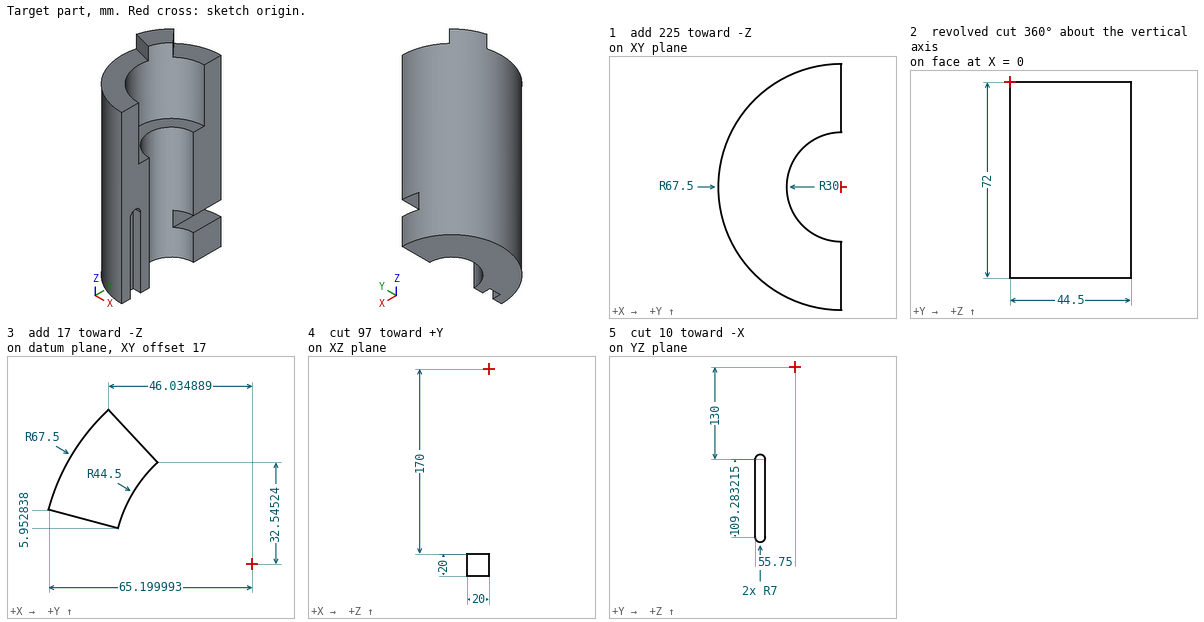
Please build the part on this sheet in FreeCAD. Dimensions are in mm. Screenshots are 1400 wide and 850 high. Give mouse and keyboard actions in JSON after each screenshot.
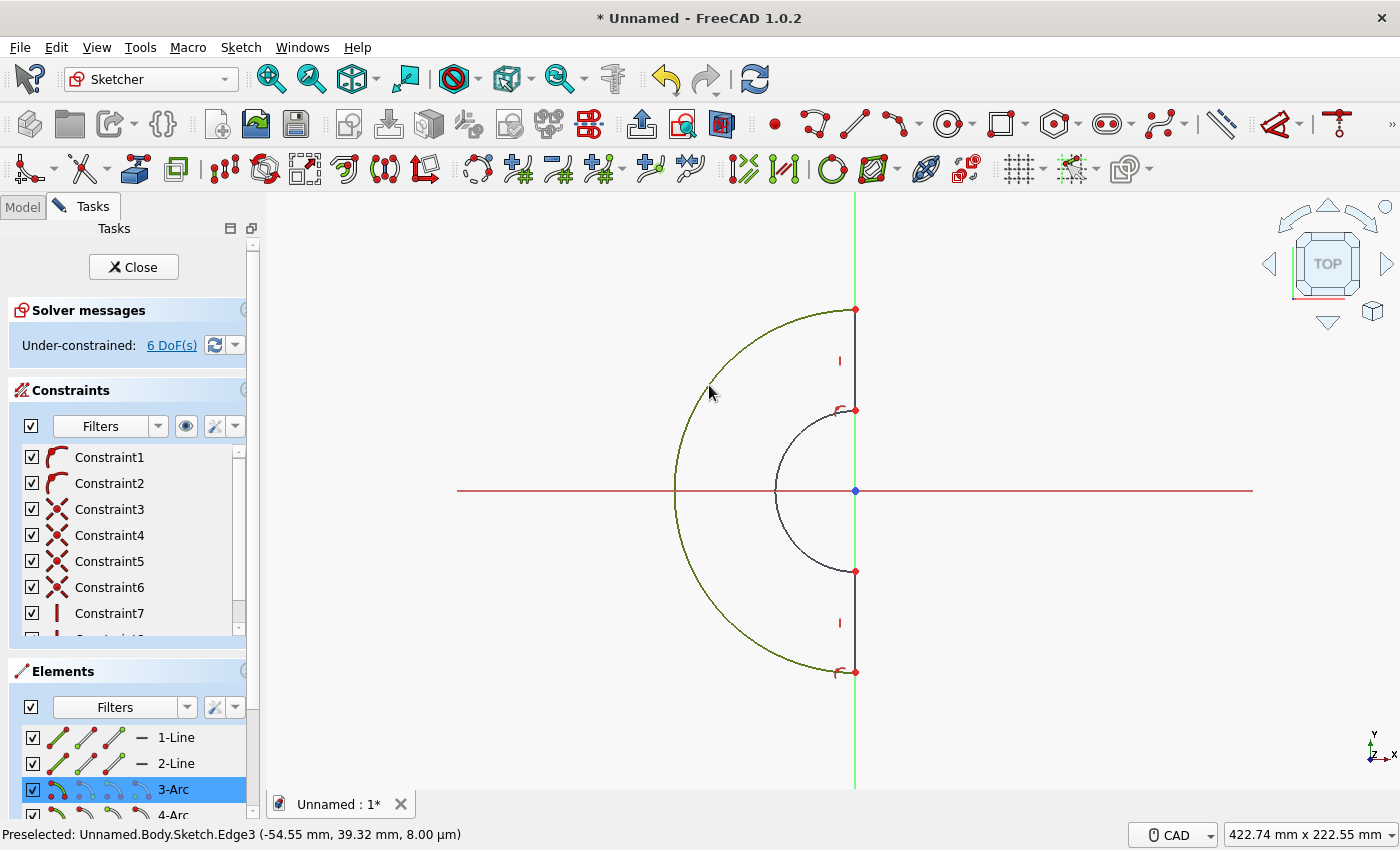
{"action": "left_click", "coordinate": [791, 444]}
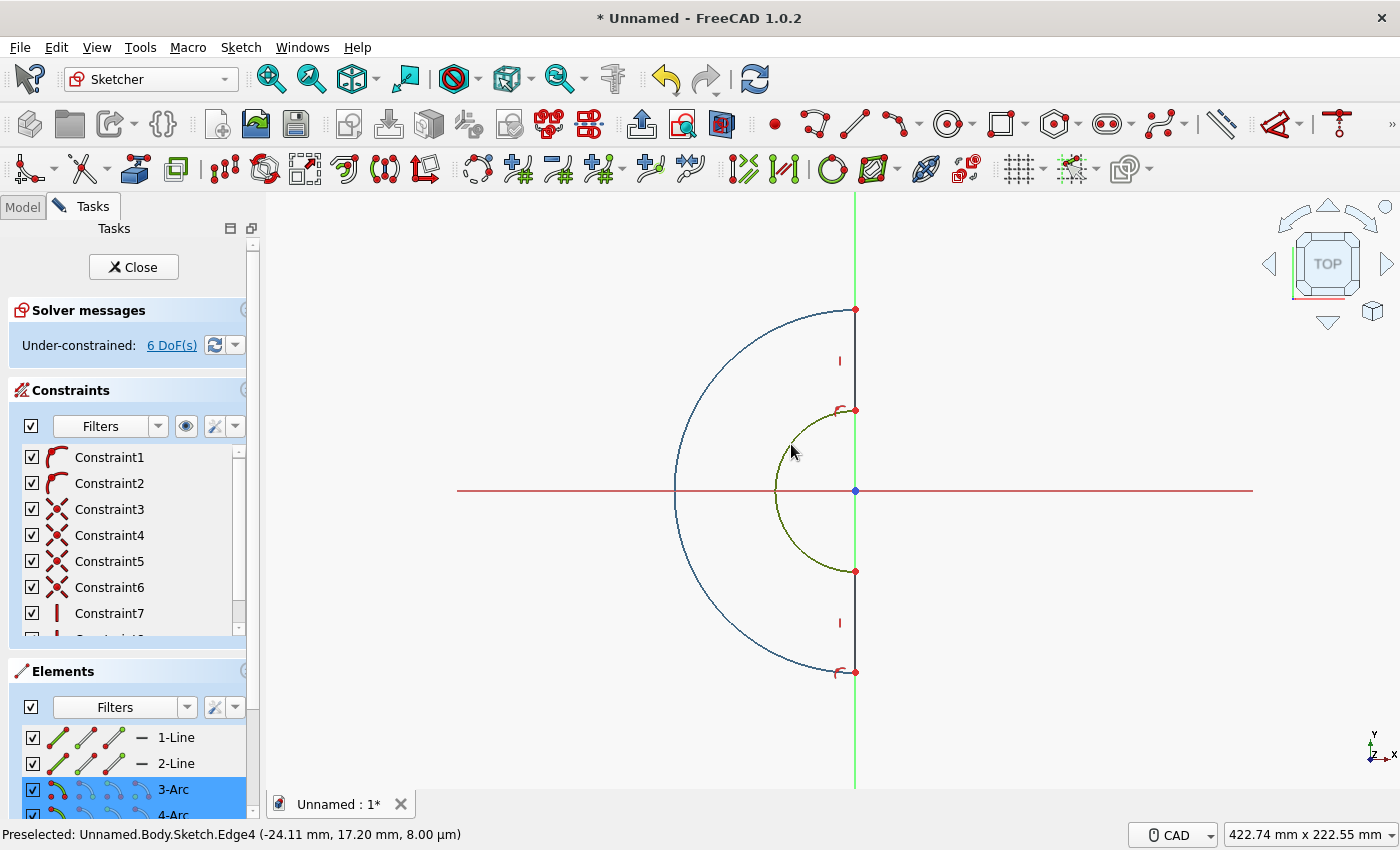
{"action": "left_click", "coordinate": [1338, 124]}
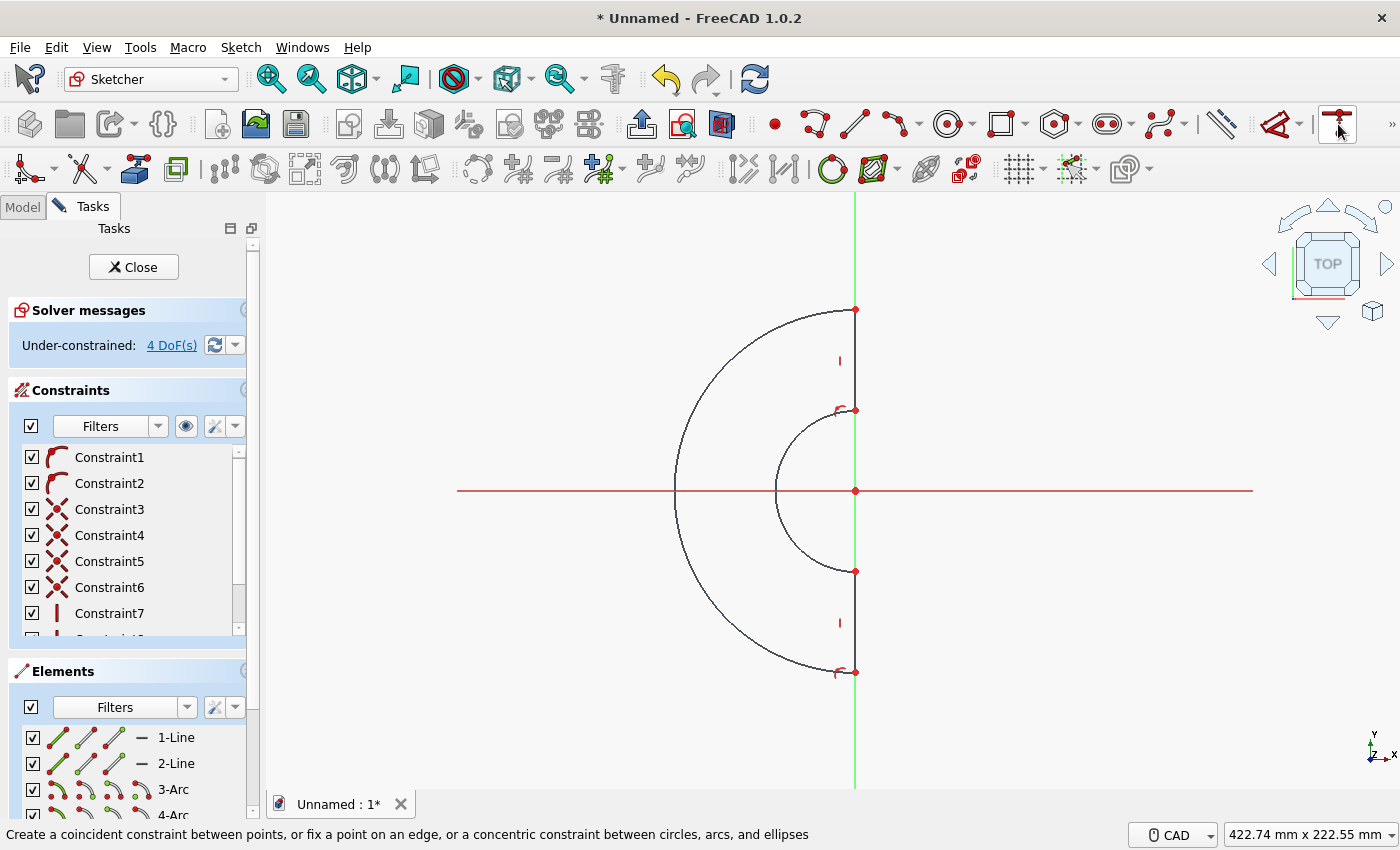
{"action": "left_click_drag", "start_coordinate": [845, 480], "coordinate": [866, 502]}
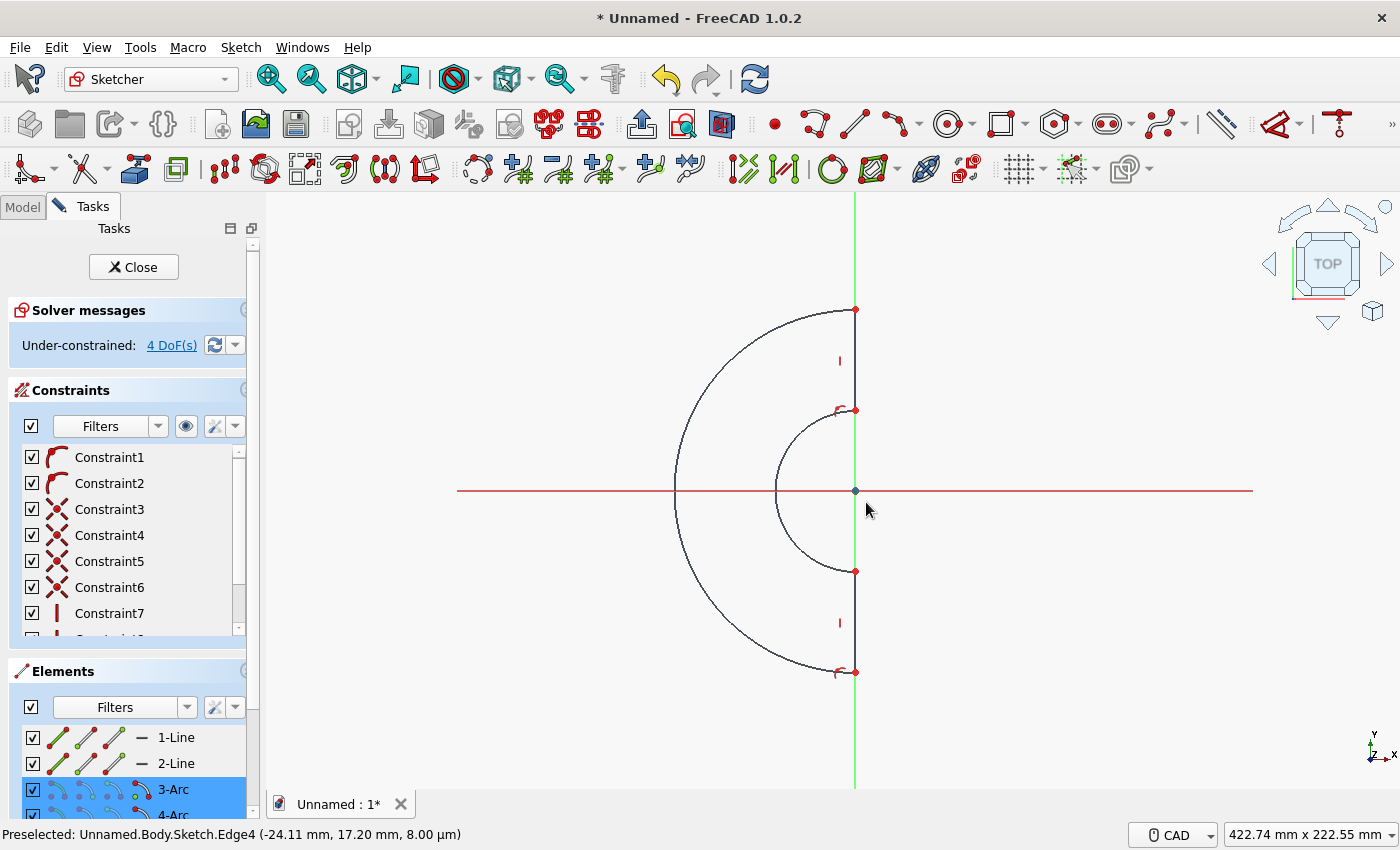
{"action": "left_click", "coordinate": [1338, 124]}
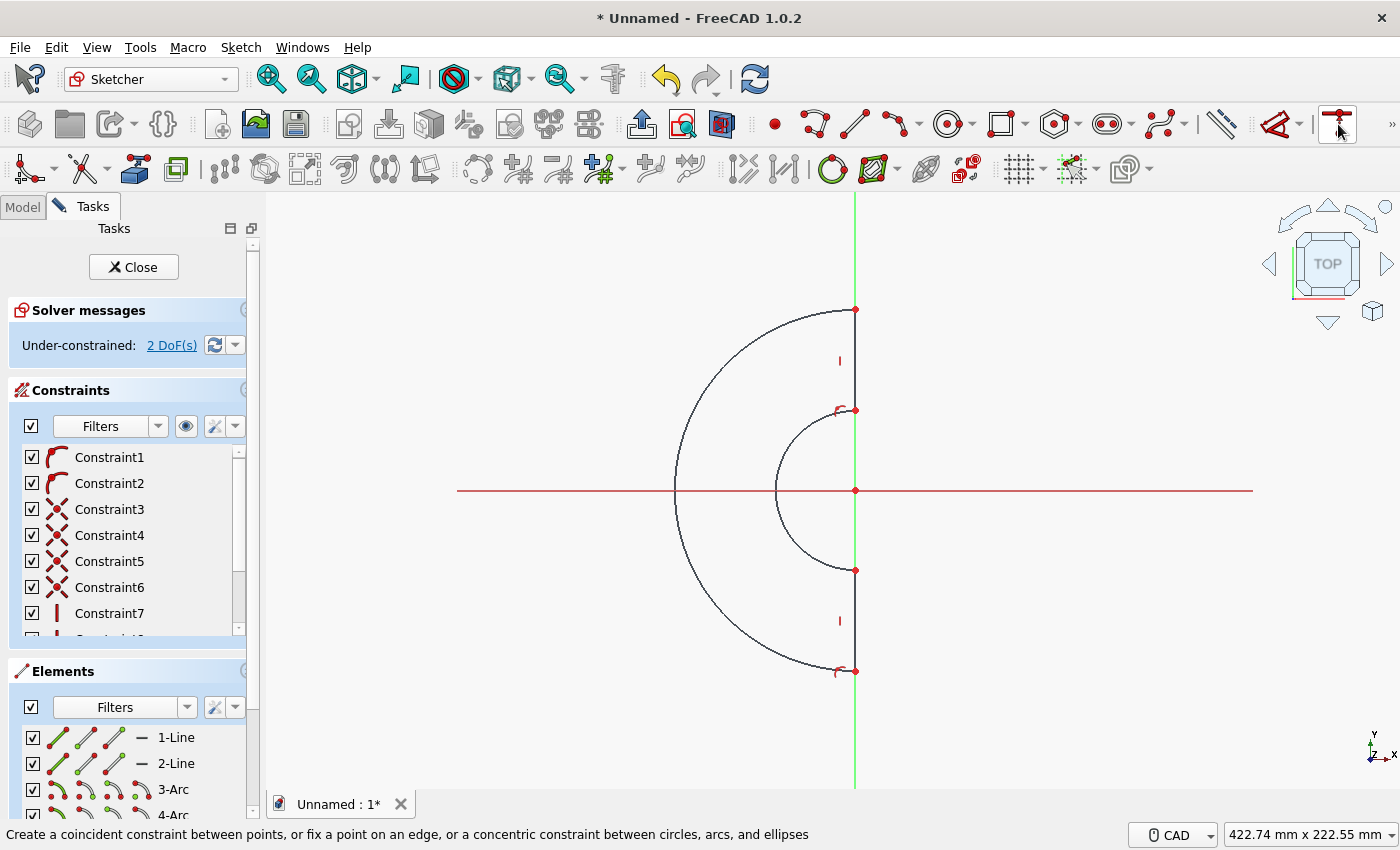
{"action": "left_click", "coordinate": [709, 384]}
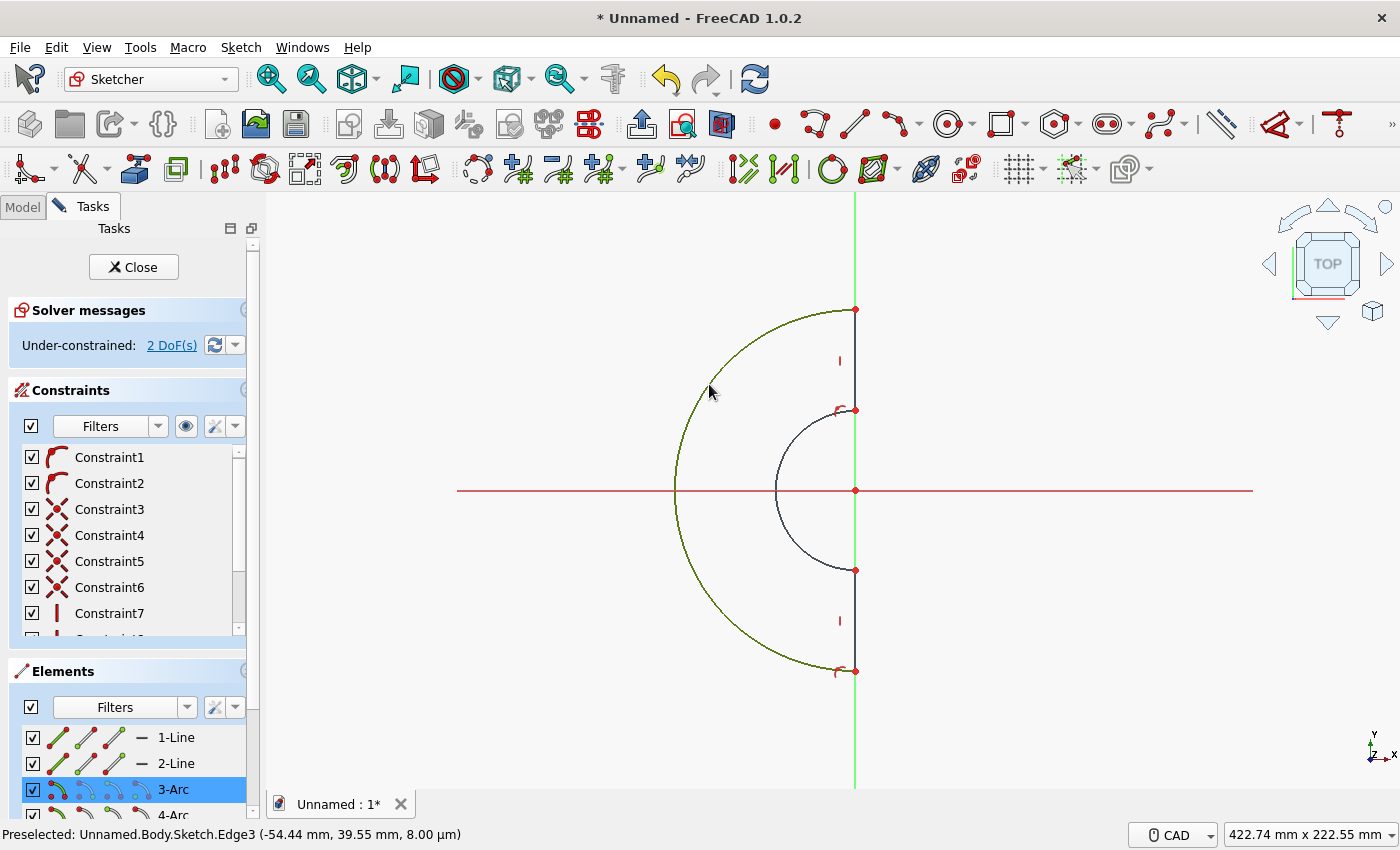
{"action": "key", "text": "k r"}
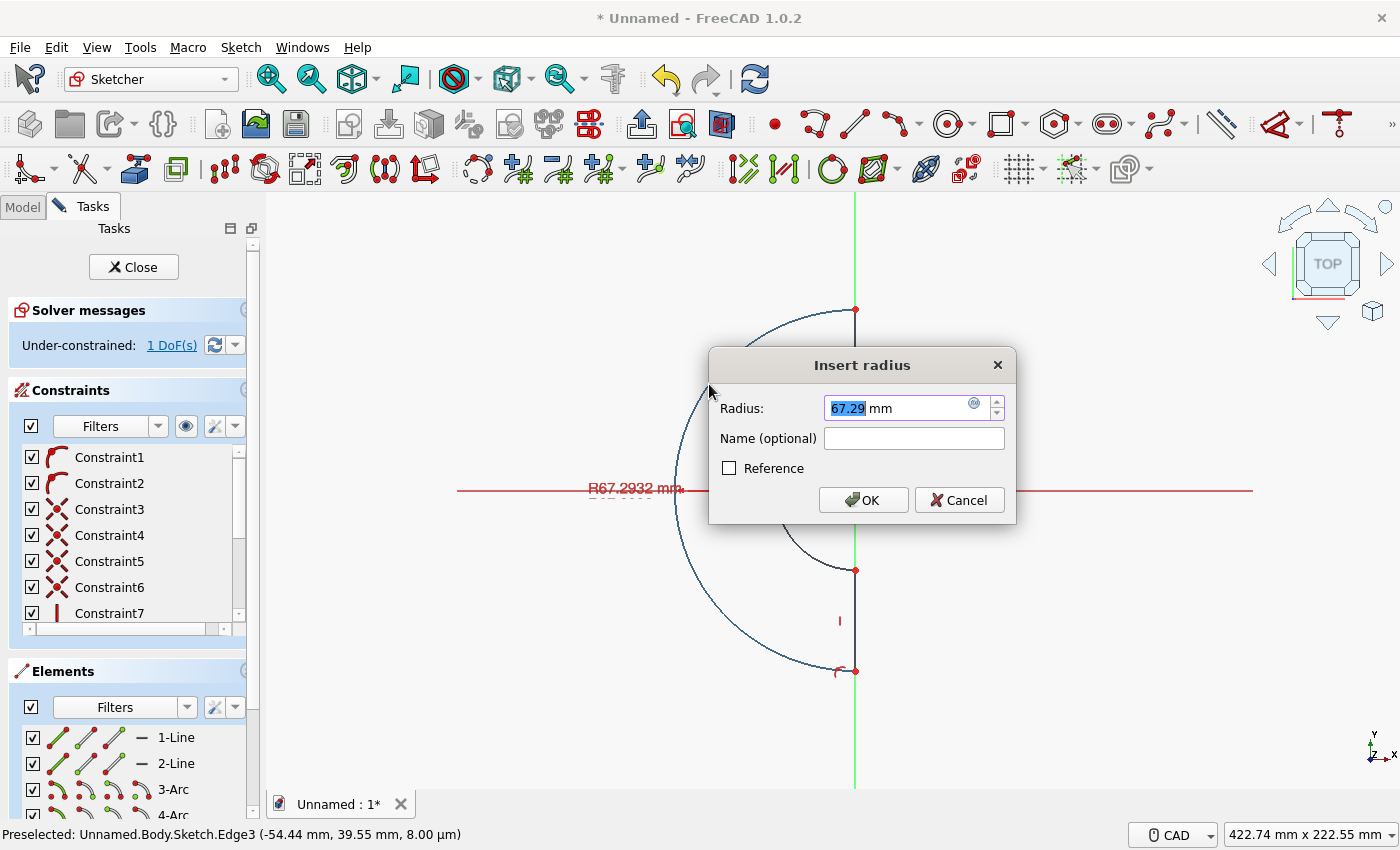
{"action": "type", "text": "67.5"}
{"action": "key", "text": "Return"}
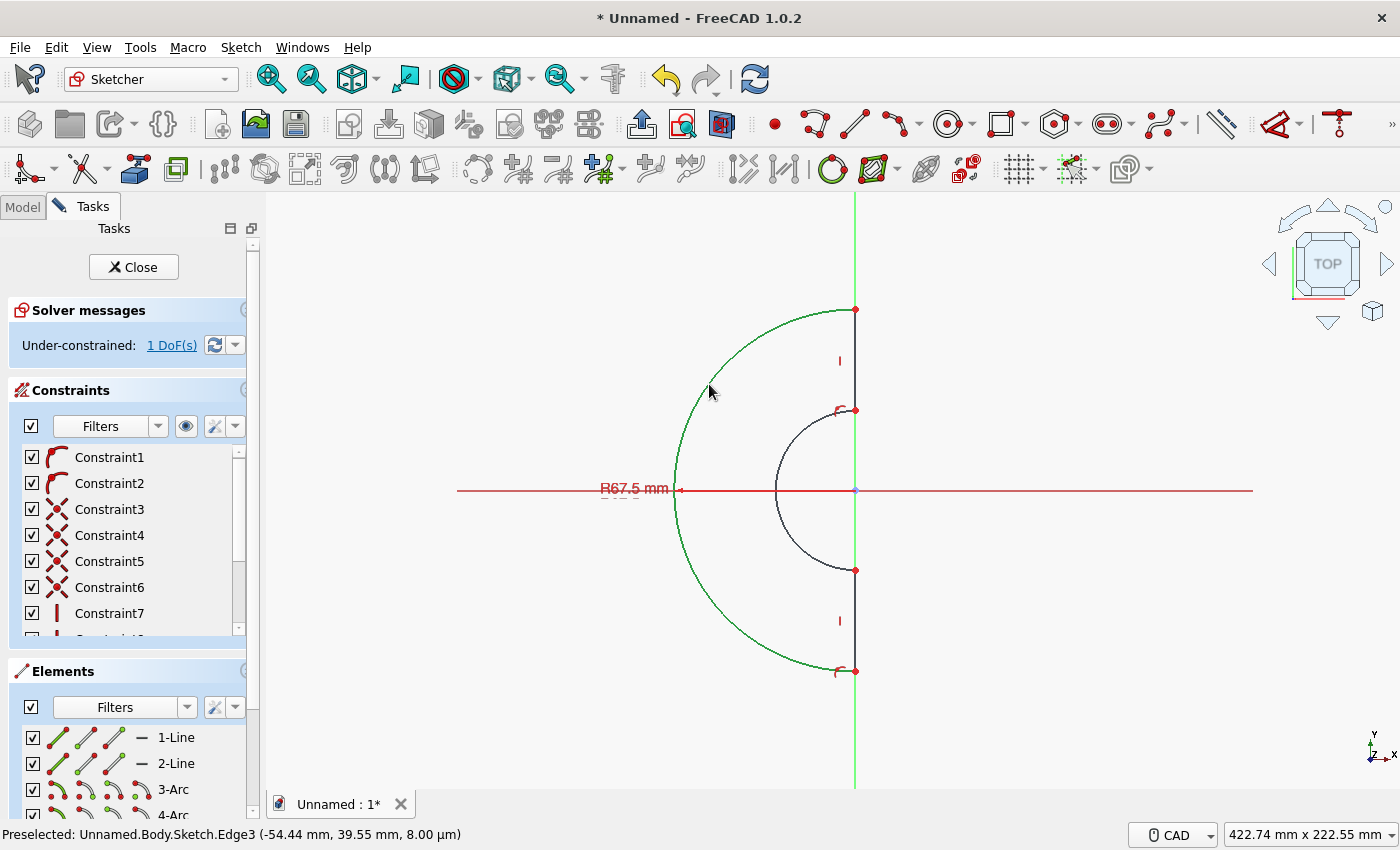
{"action": "left_click", "coordinate": [791, 444]}